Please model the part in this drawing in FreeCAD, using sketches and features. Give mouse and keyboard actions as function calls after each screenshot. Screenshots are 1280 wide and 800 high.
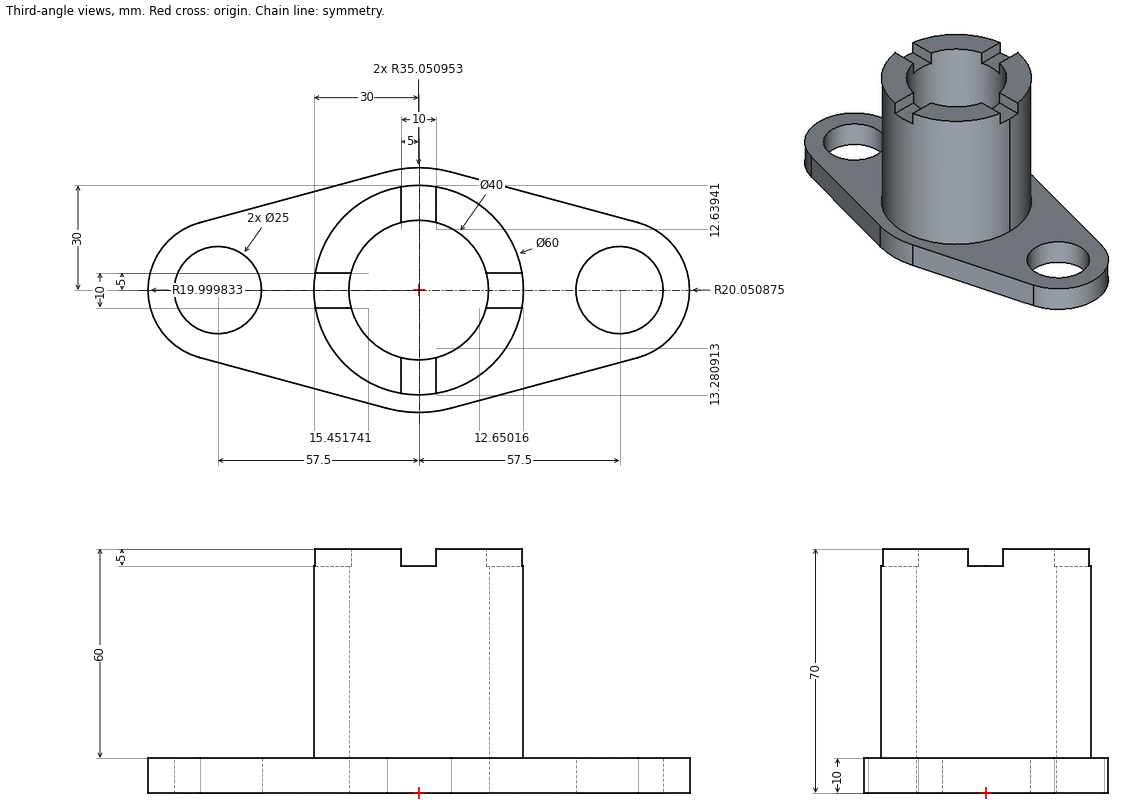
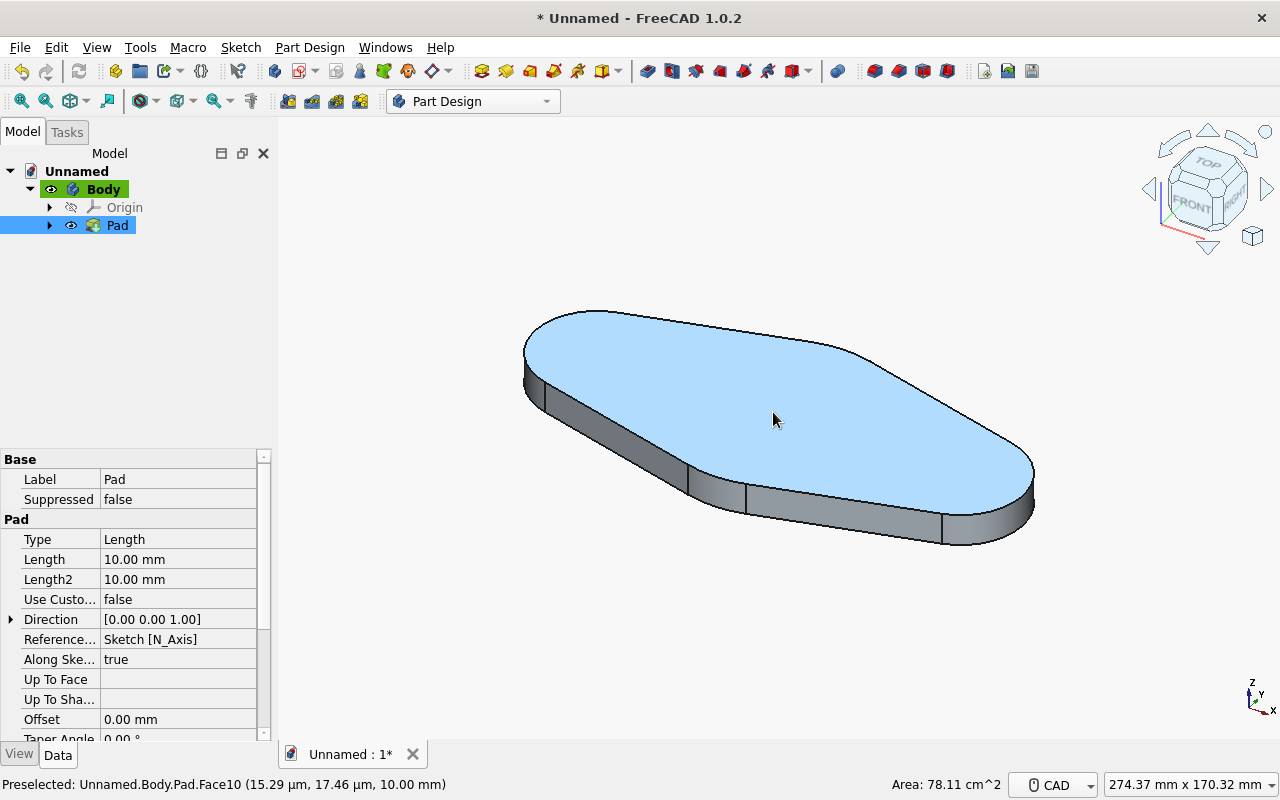
click(300, 72)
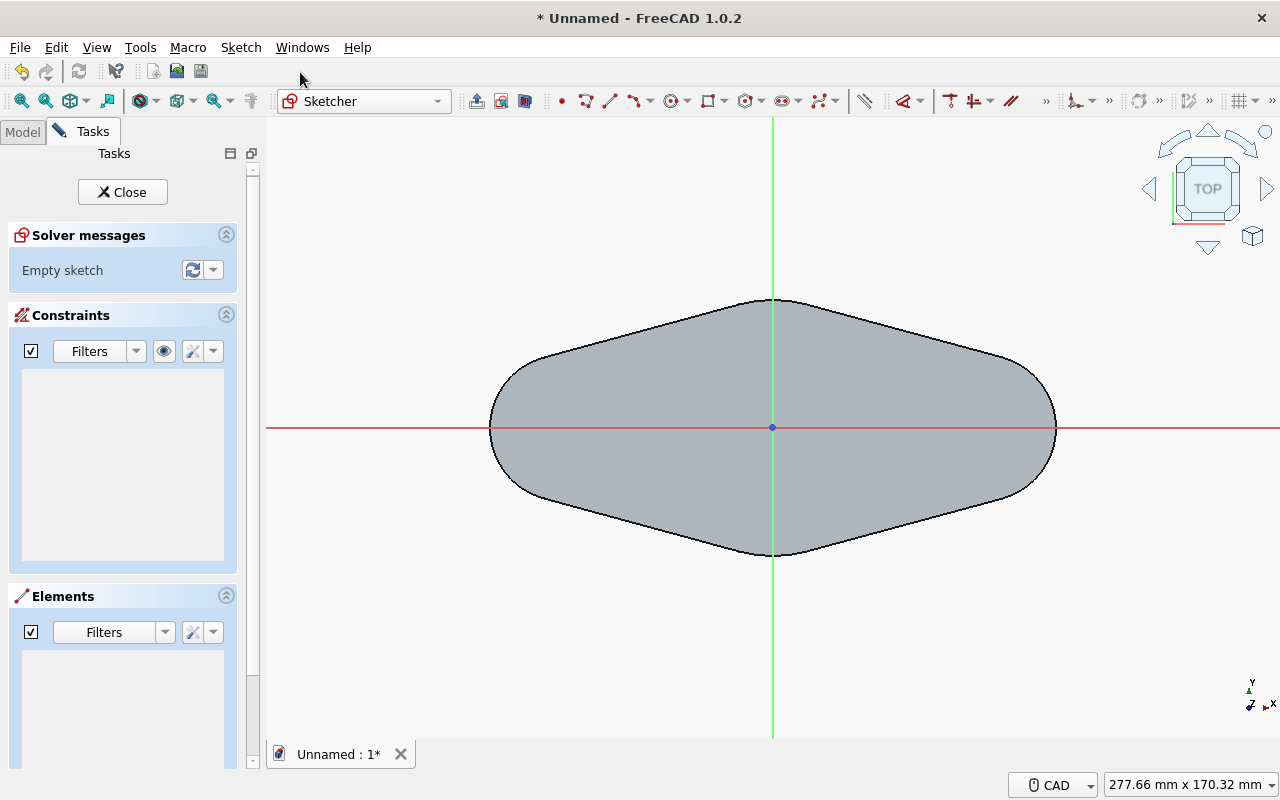
scroll(856, 428, up, 3)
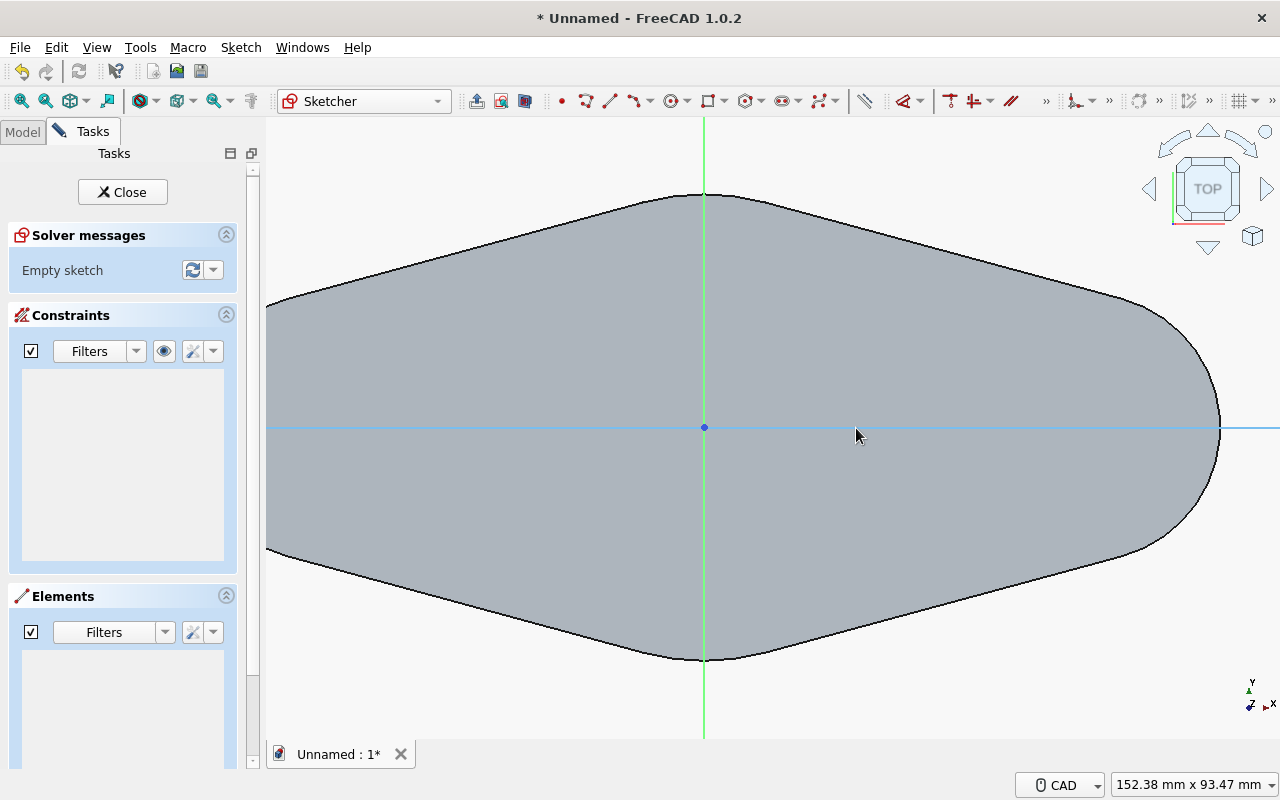
key(g)
key(c)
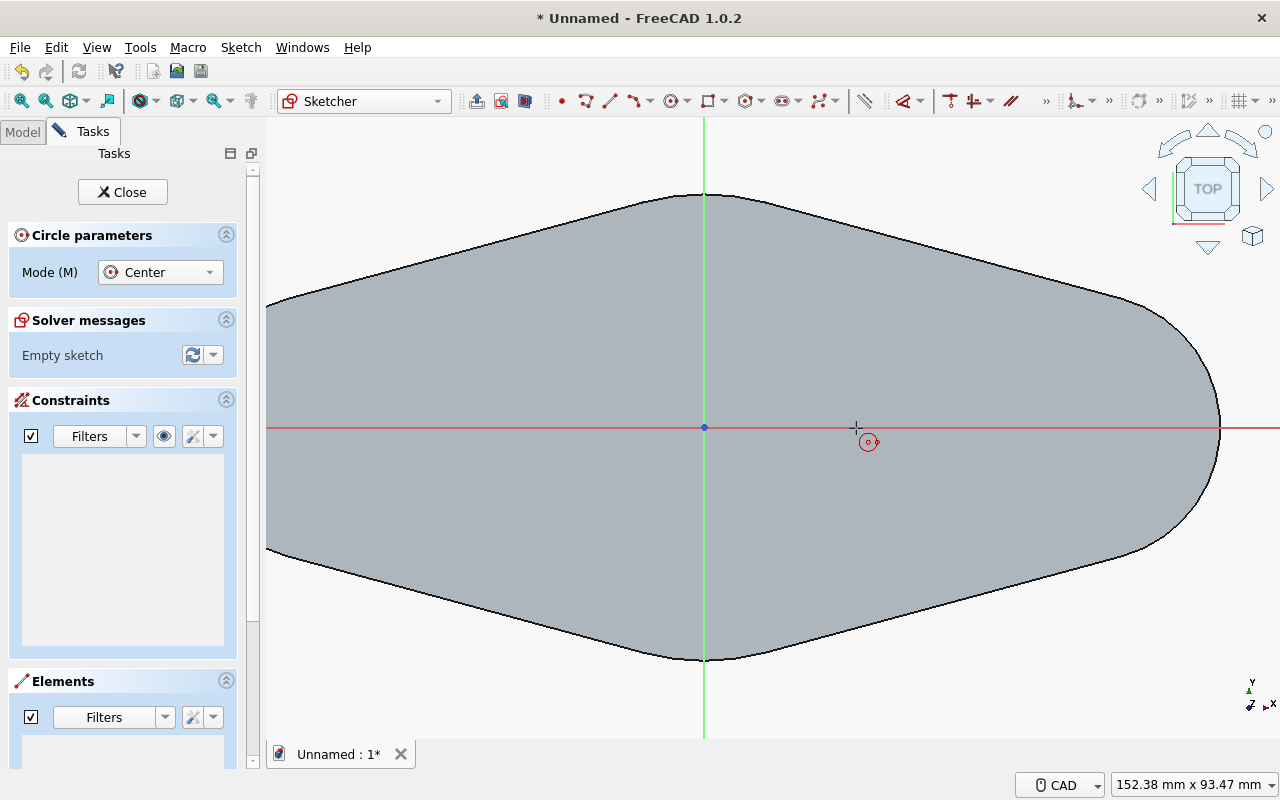
click(704, 428)
move(845, 286)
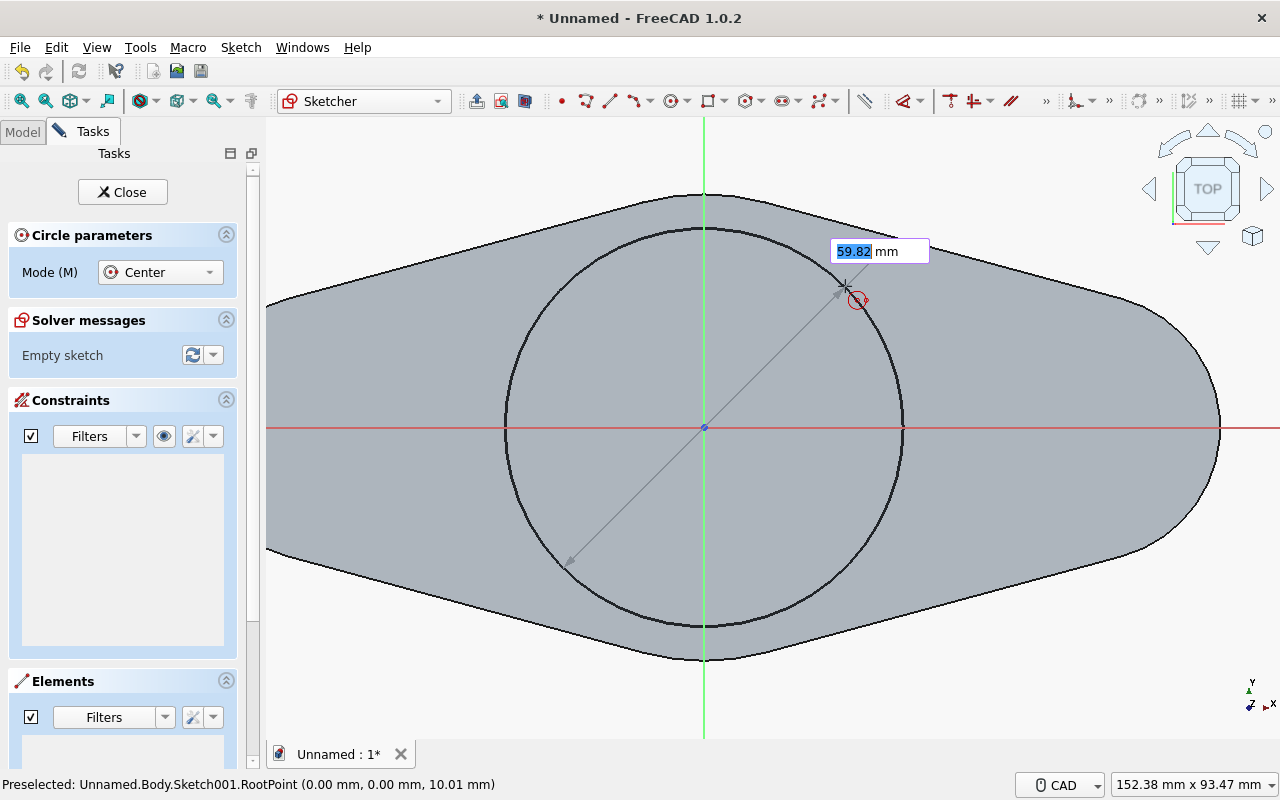
text(60)
key(Return)
key(Escape)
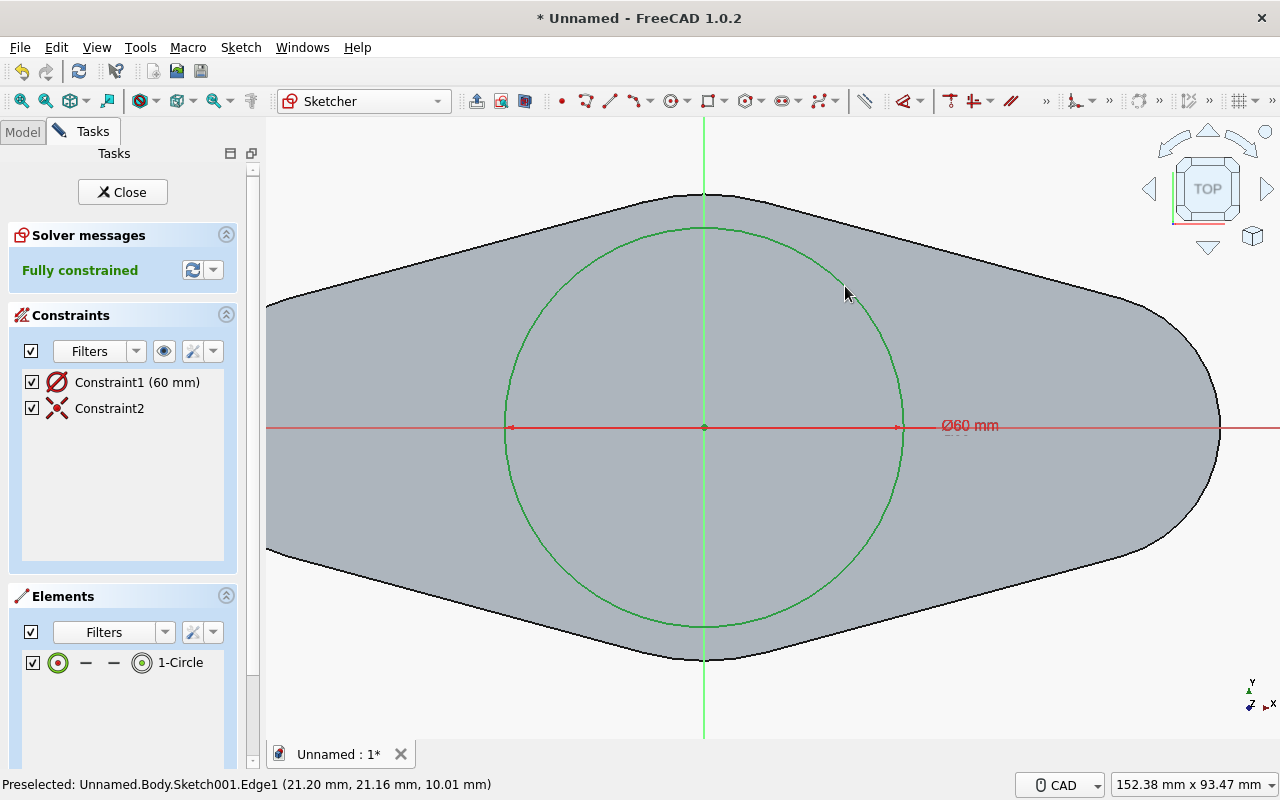
click(123, 192)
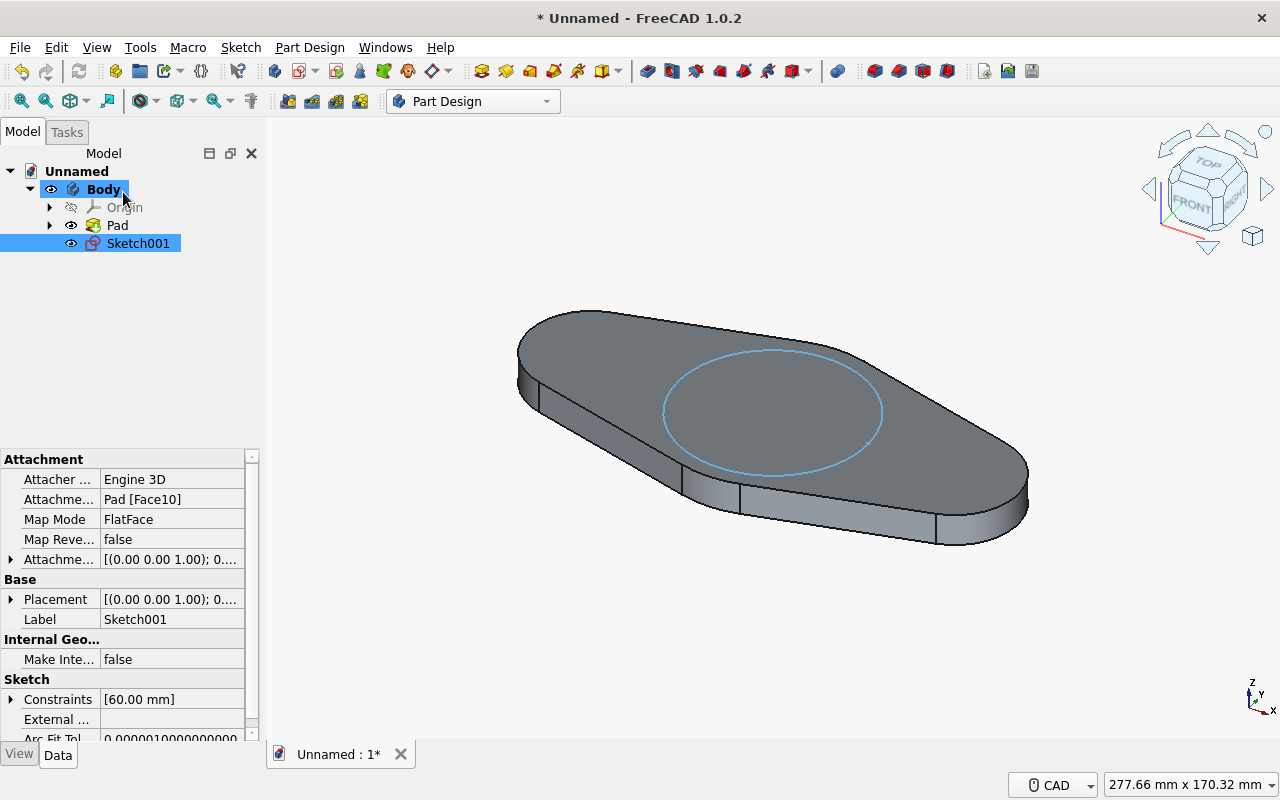
click(482, 72)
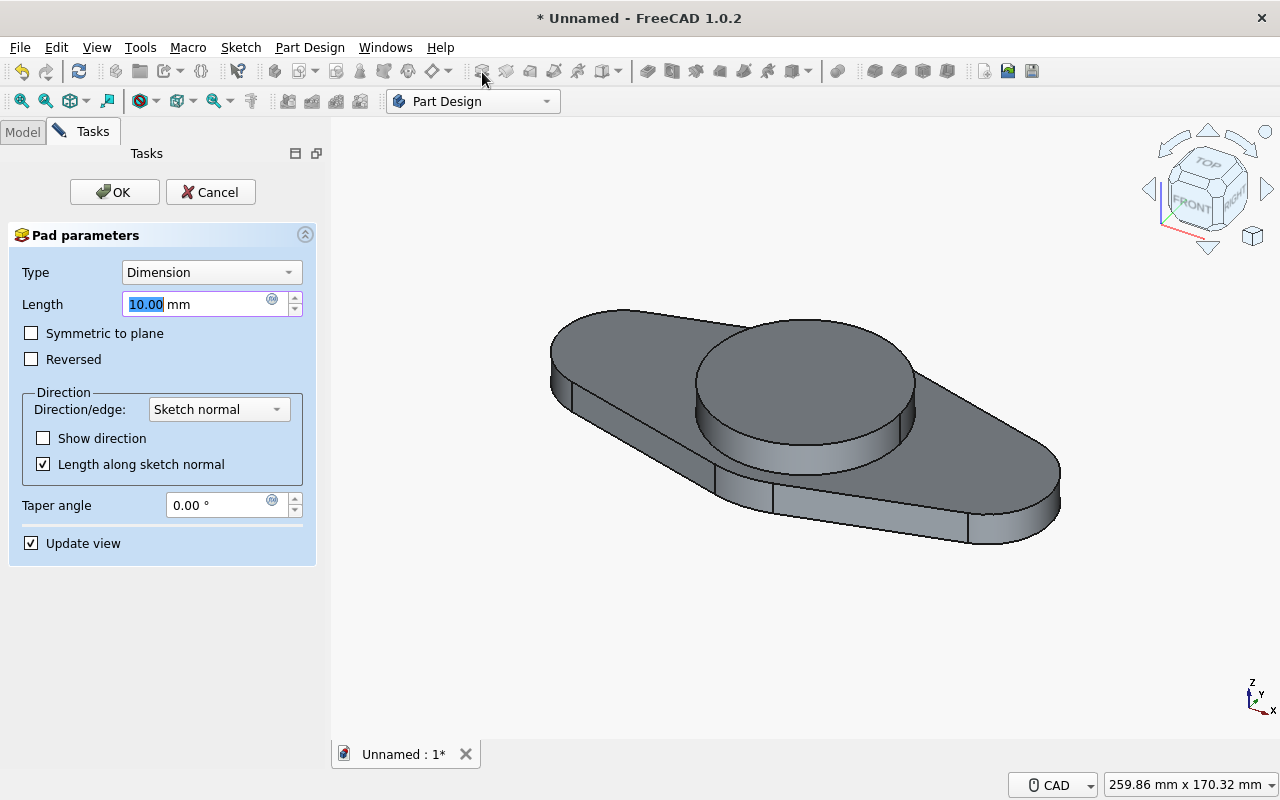
text(60)
key(Tab)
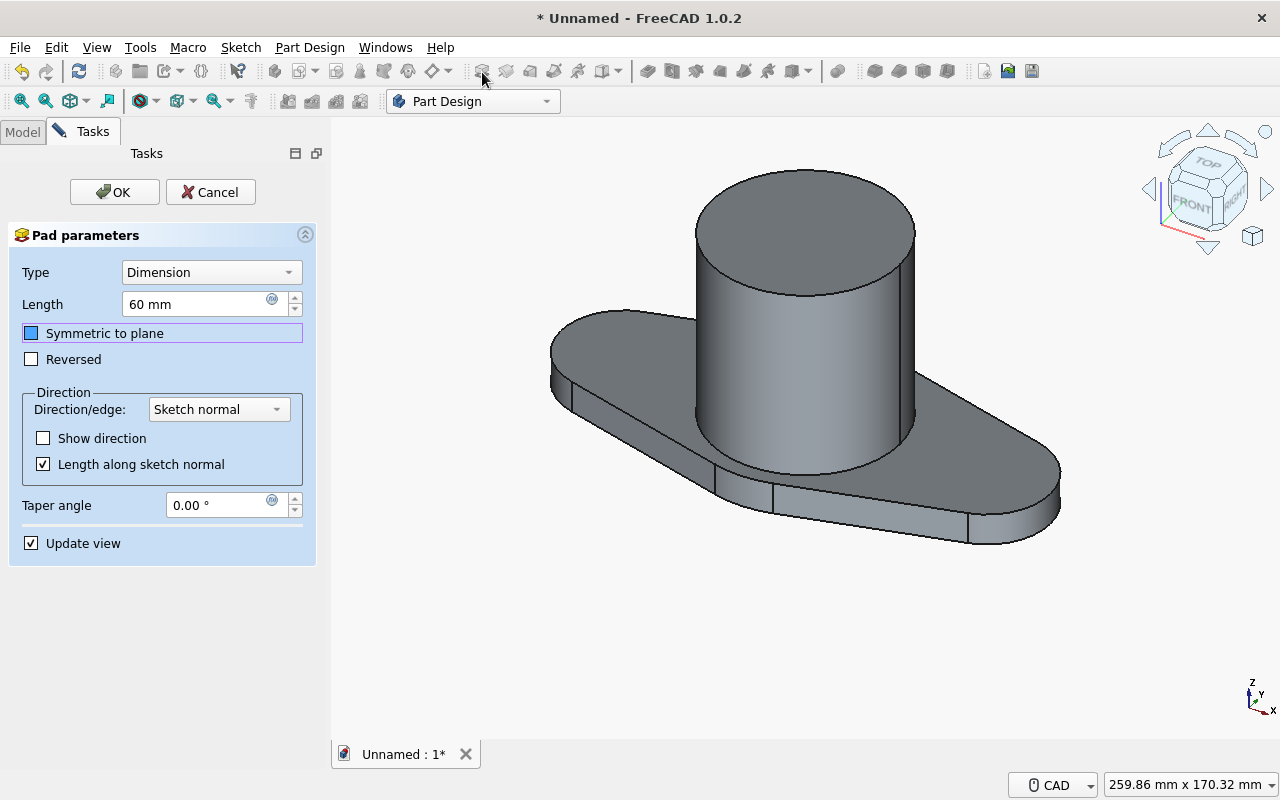
click(115, 192)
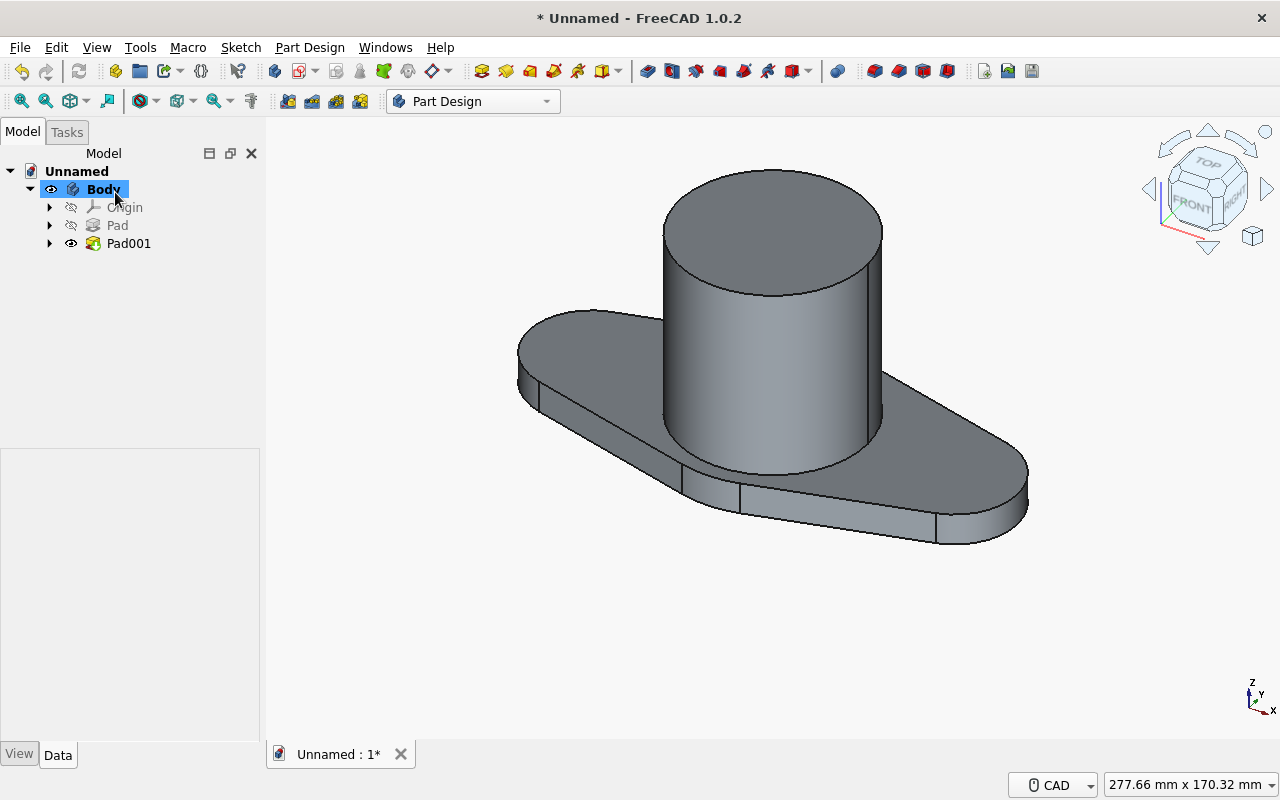
click(22, 102)